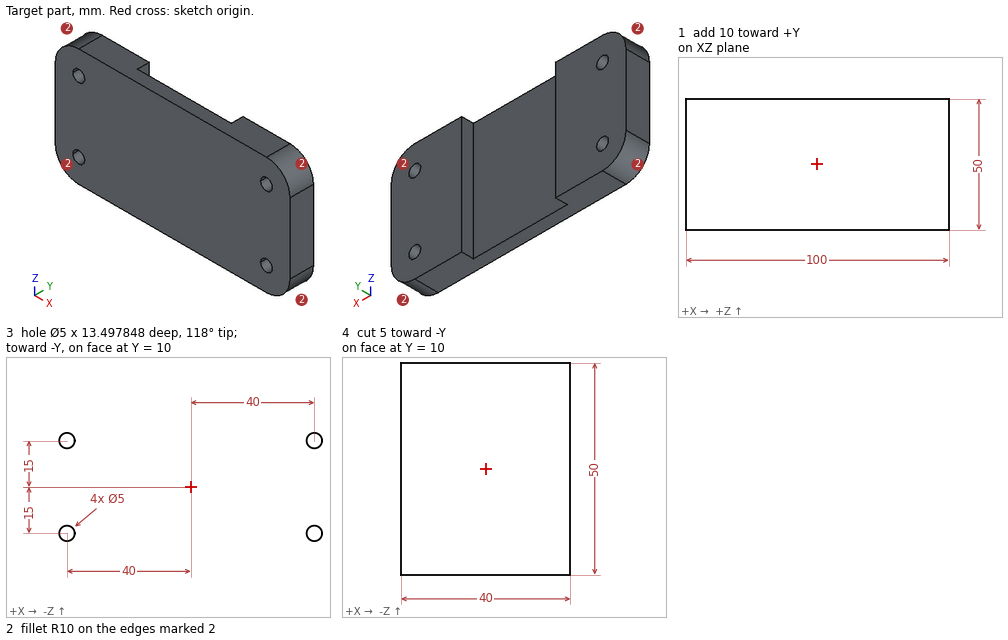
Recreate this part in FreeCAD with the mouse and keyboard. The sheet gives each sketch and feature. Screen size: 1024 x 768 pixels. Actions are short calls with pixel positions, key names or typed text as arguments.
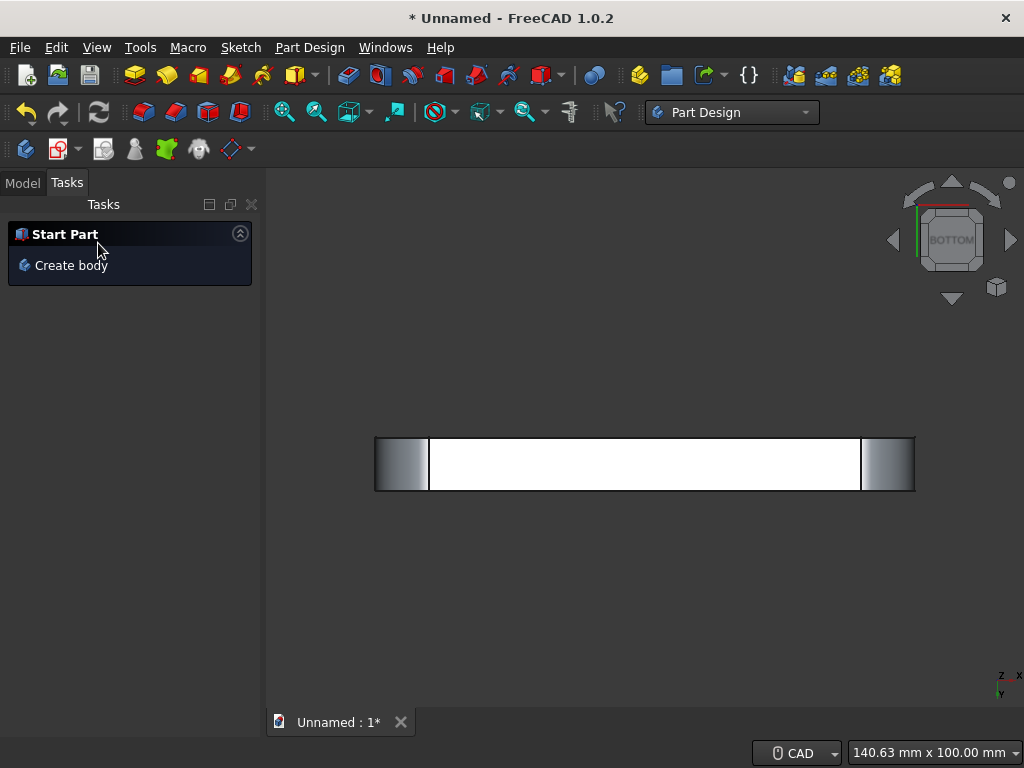
key(4)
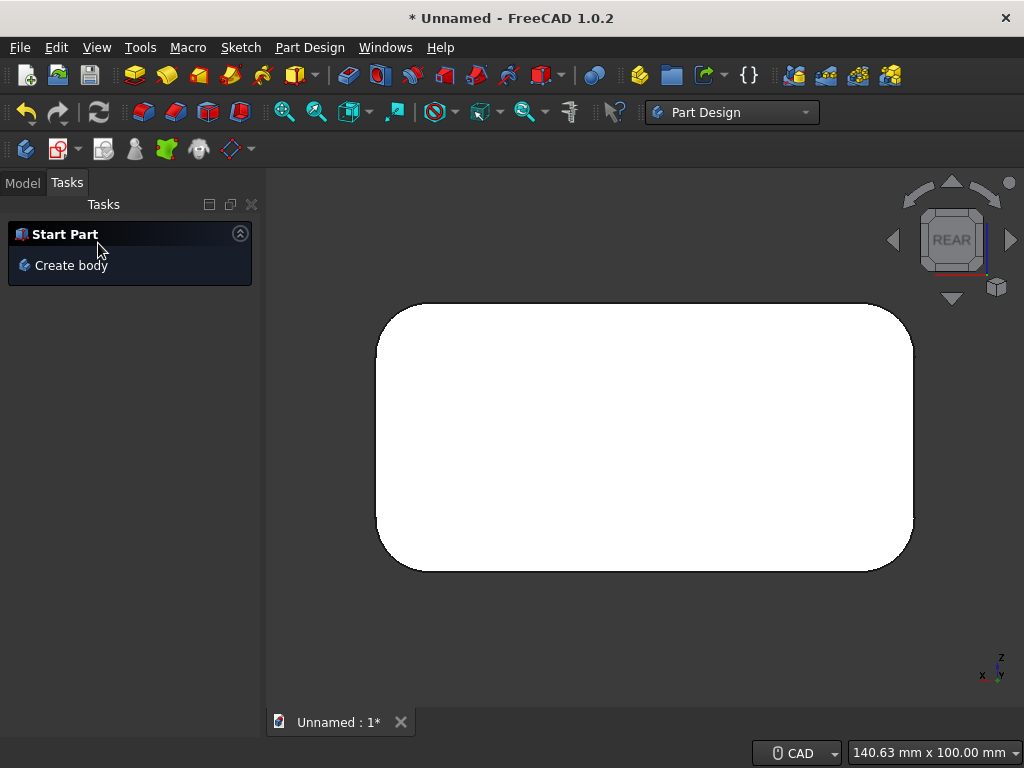
click(568, 436)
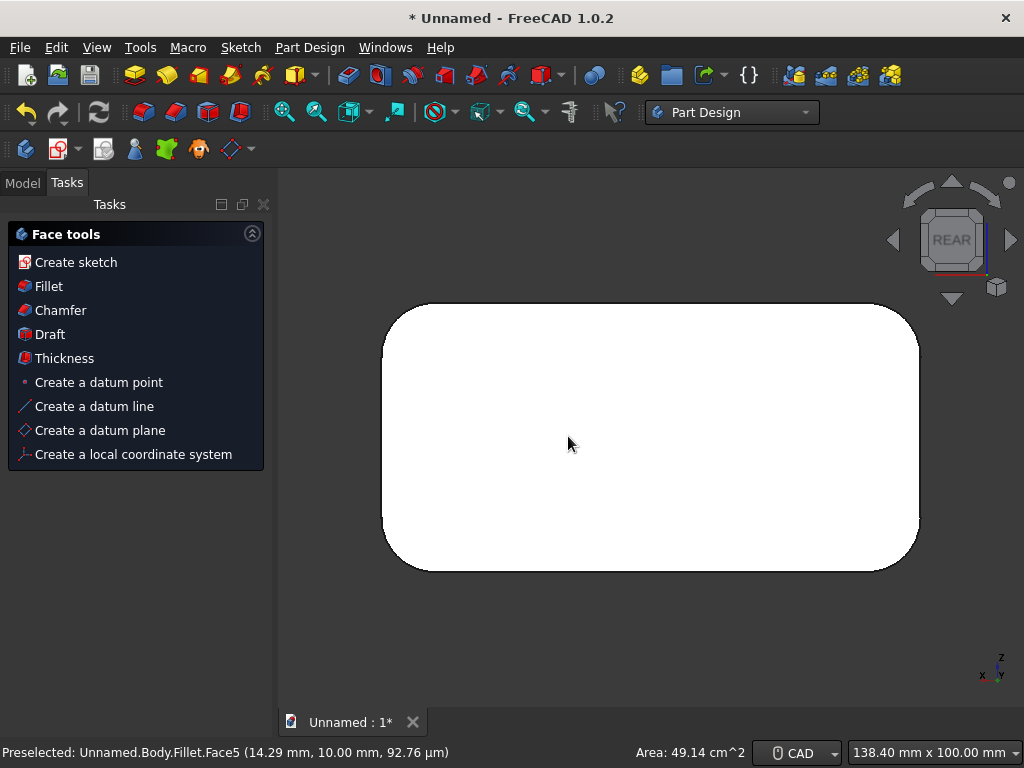
click(58, 150)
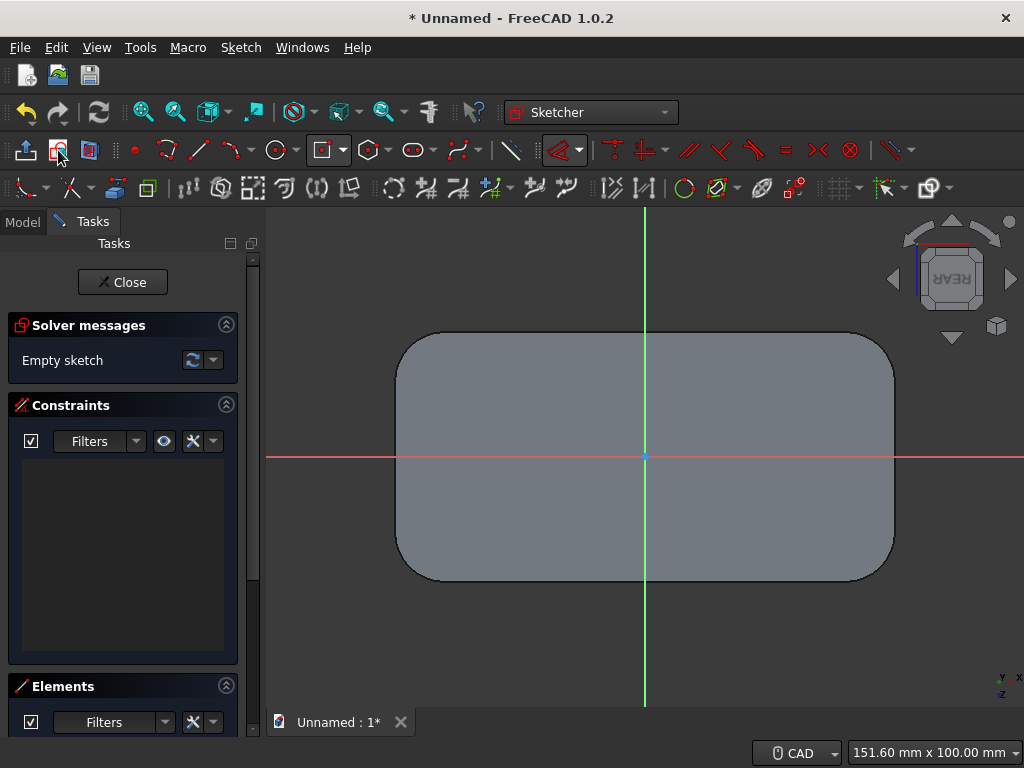
scroll(294, 457, down, 1)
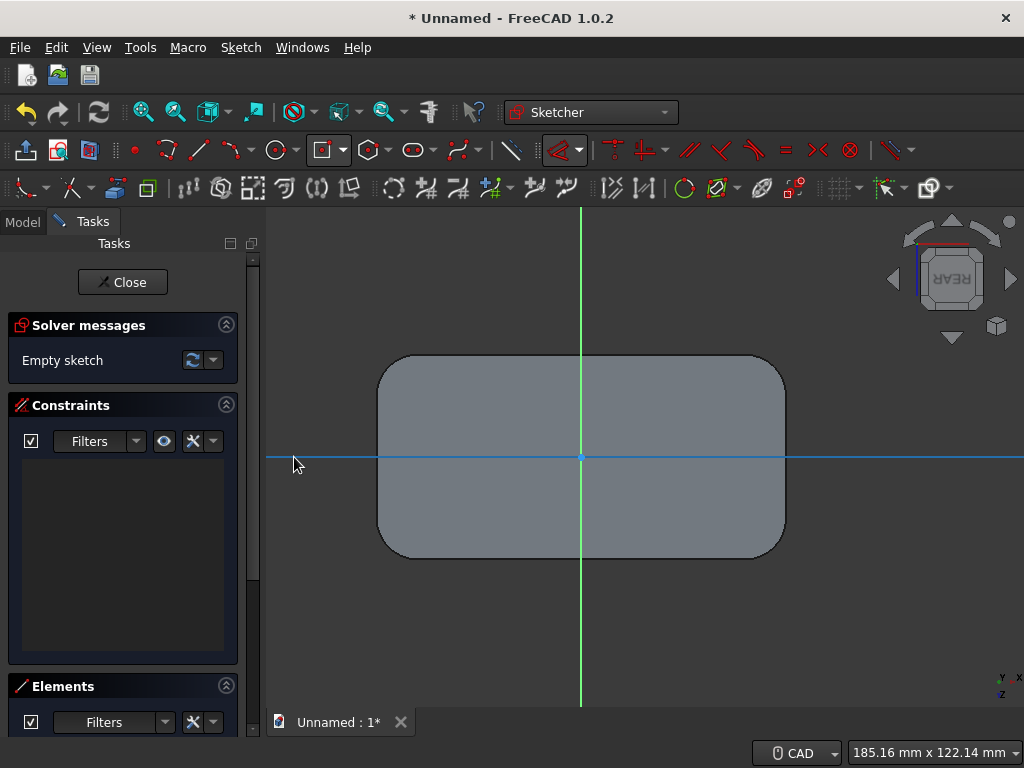
key(g)
key(c)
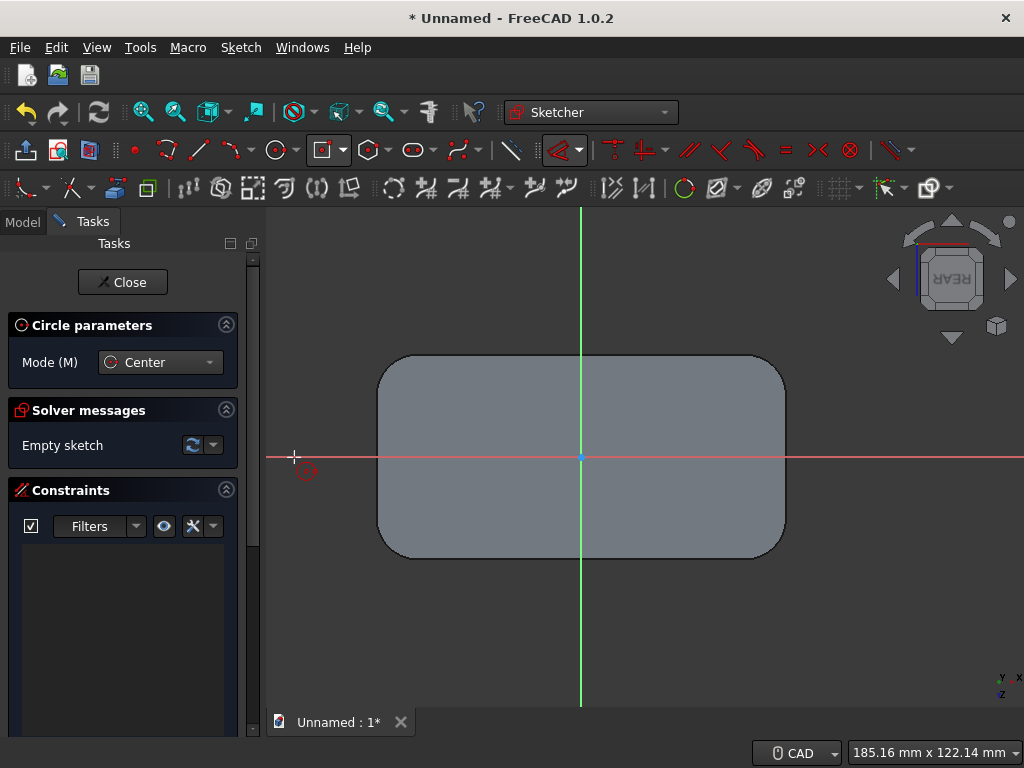
scroll(418, 518, up, 4)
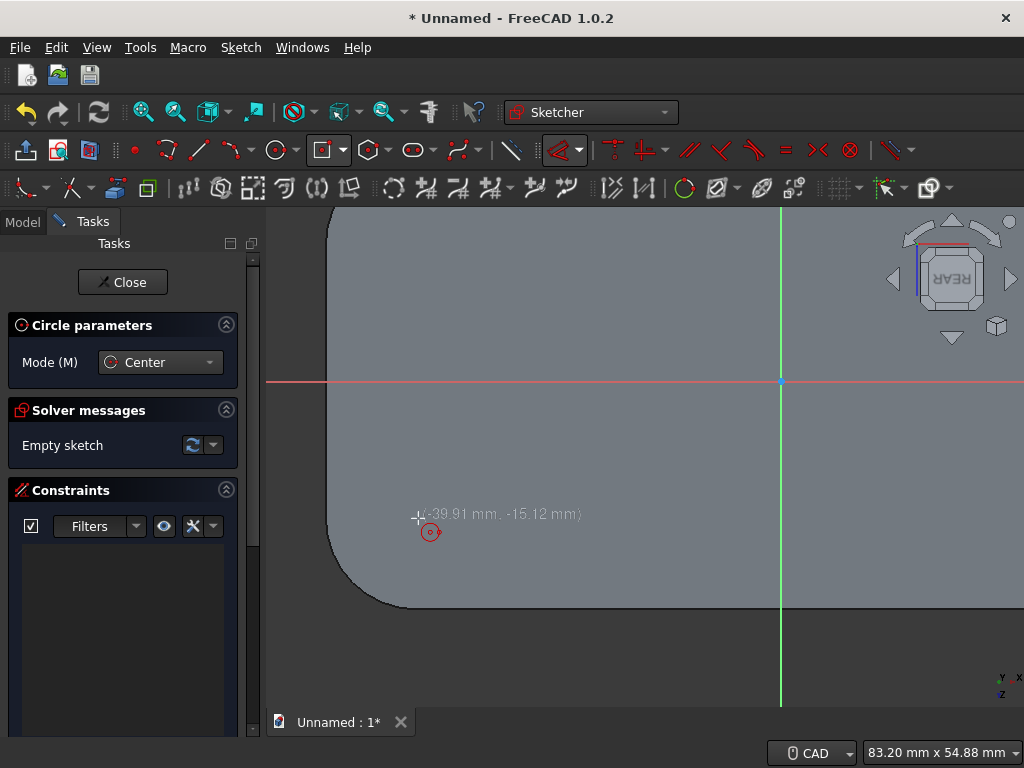
click(417, 518)
move(433, 502)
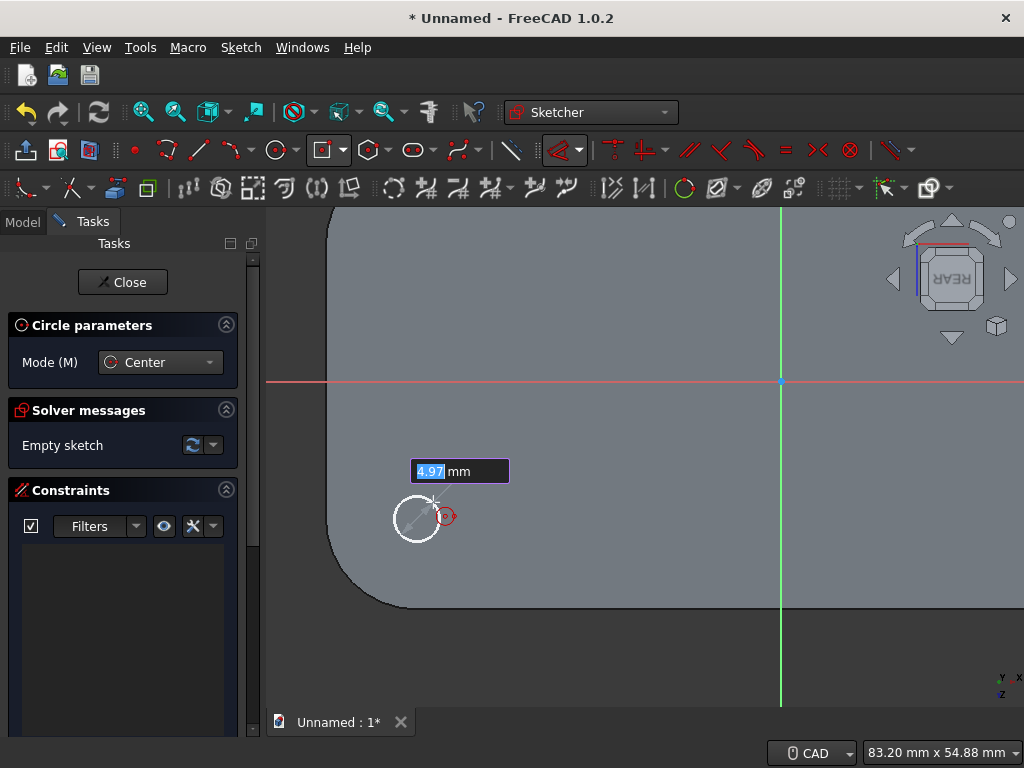
text(5)
key(Return)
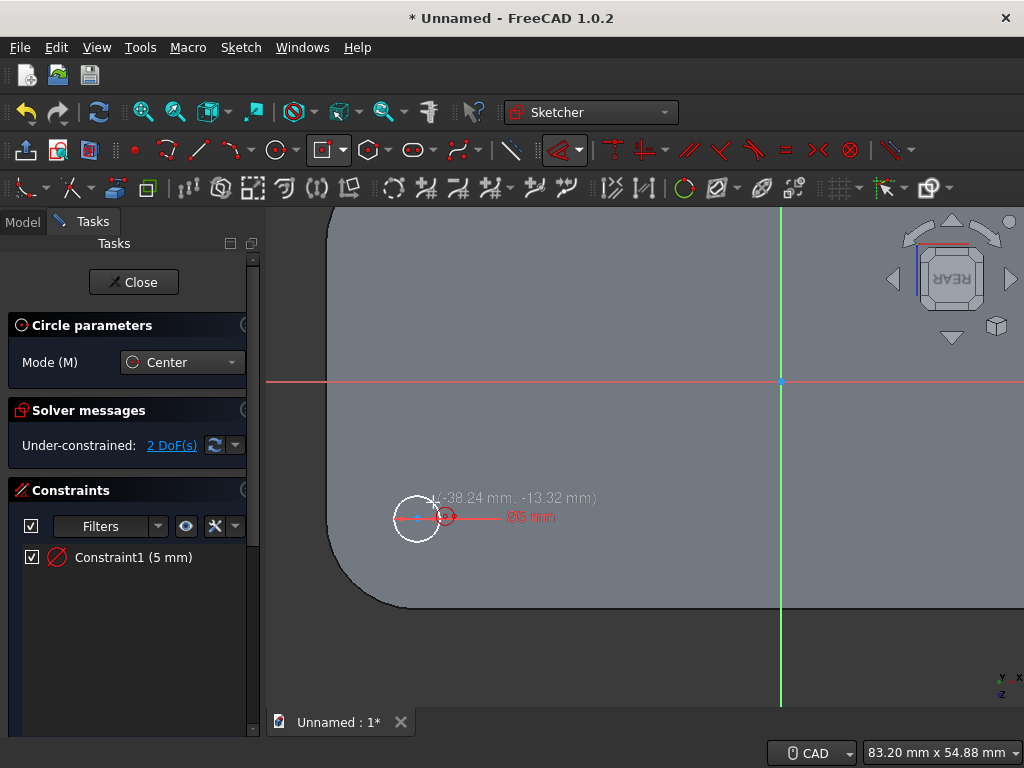
click(417, 245)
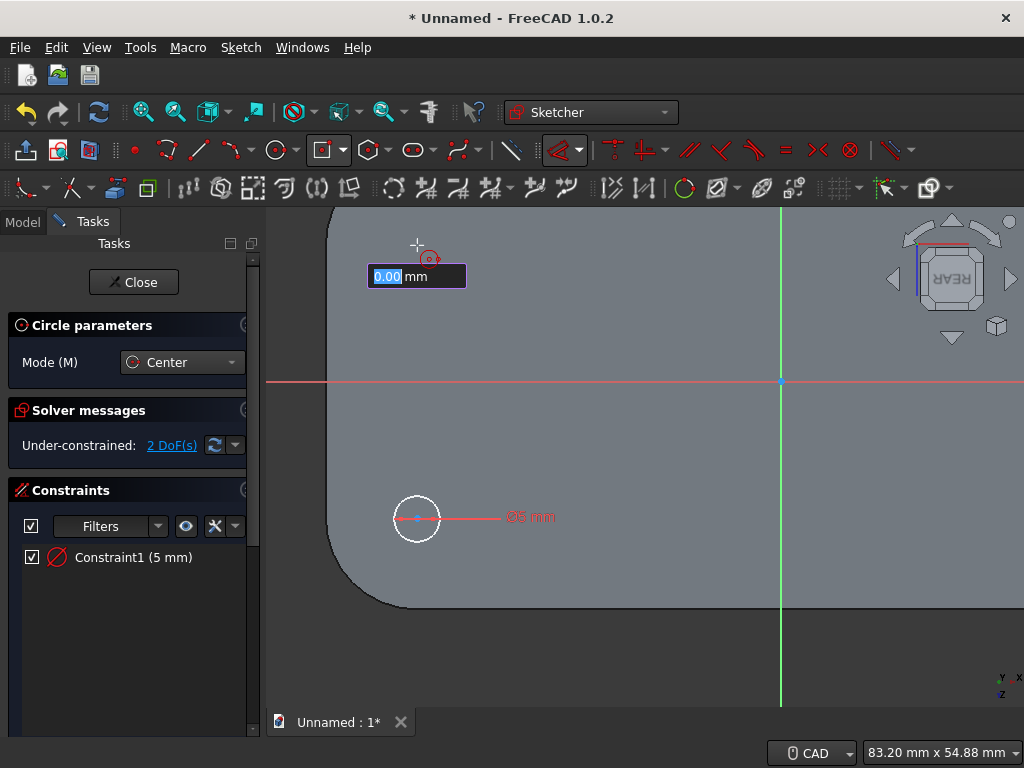
scroll(327, 549, down, 3)
move(385, 374)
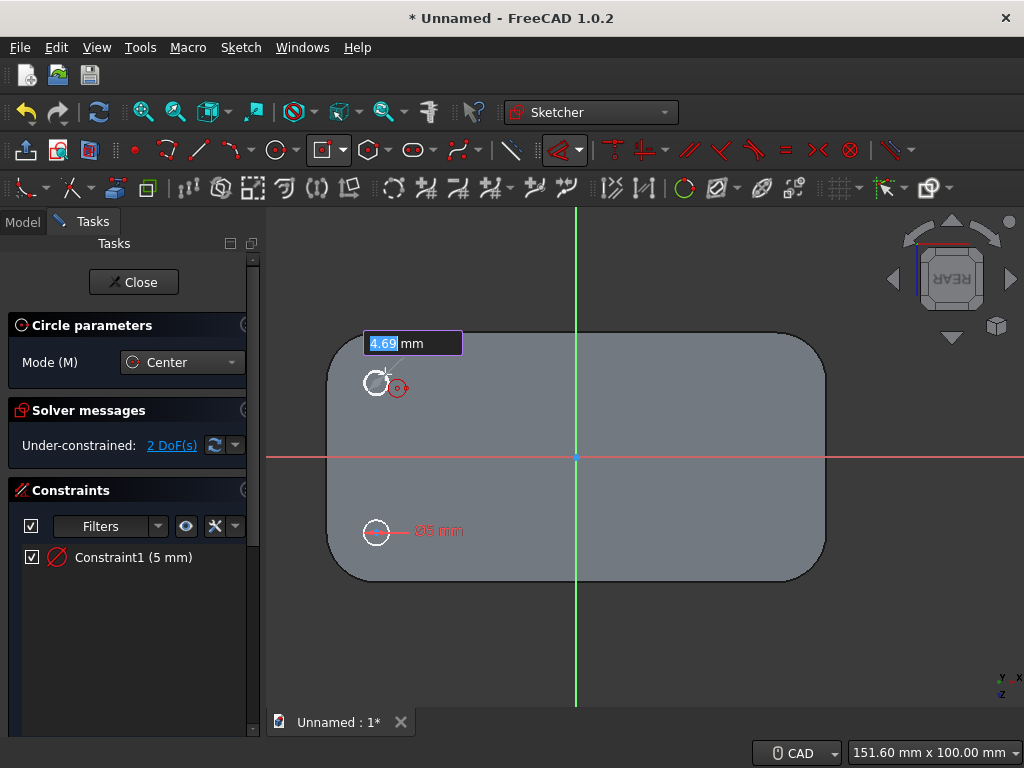
text(5)
key(Return)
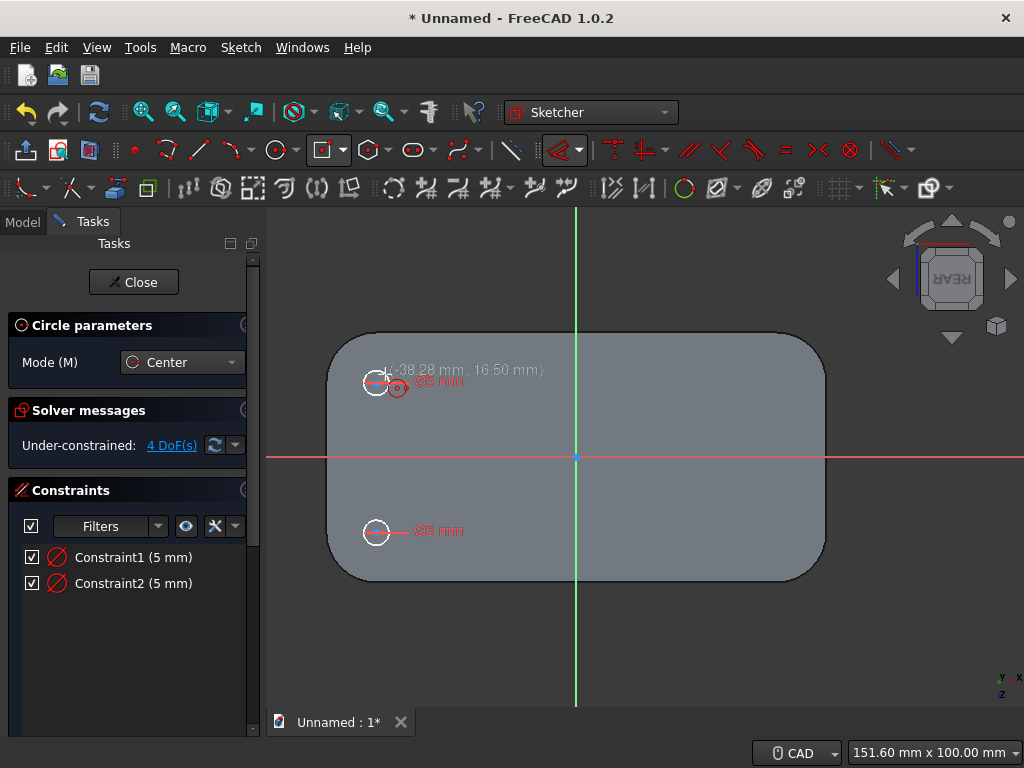
scroll(776, 382, up, 3)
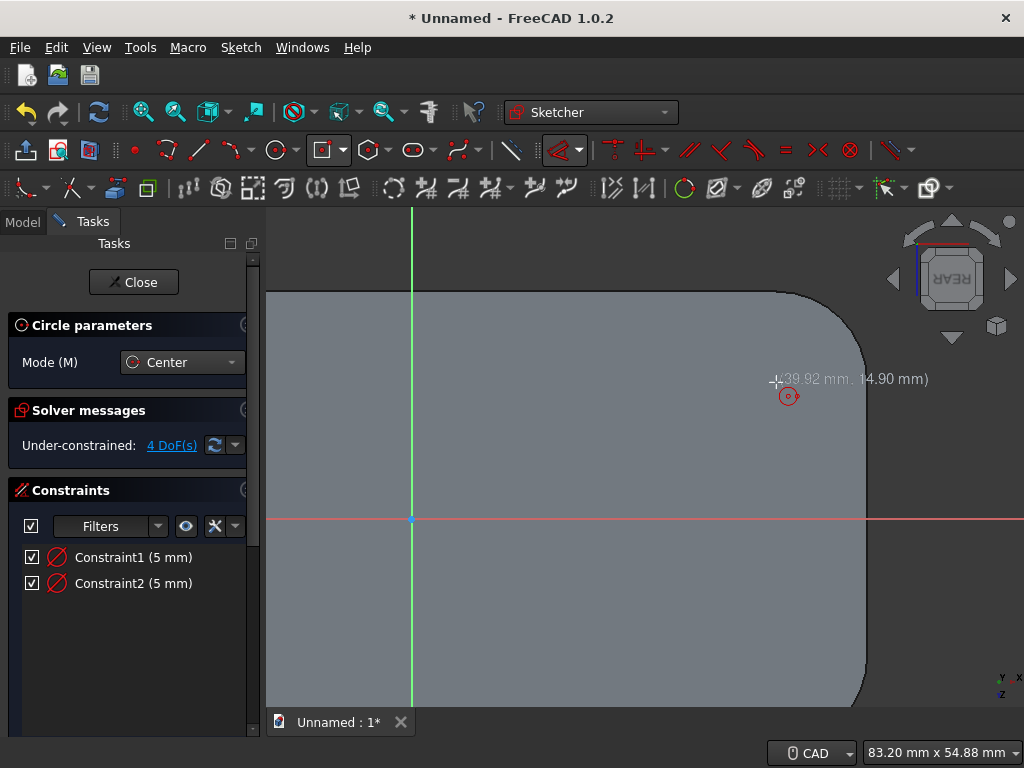
click(776, 383)
move(792, 366)